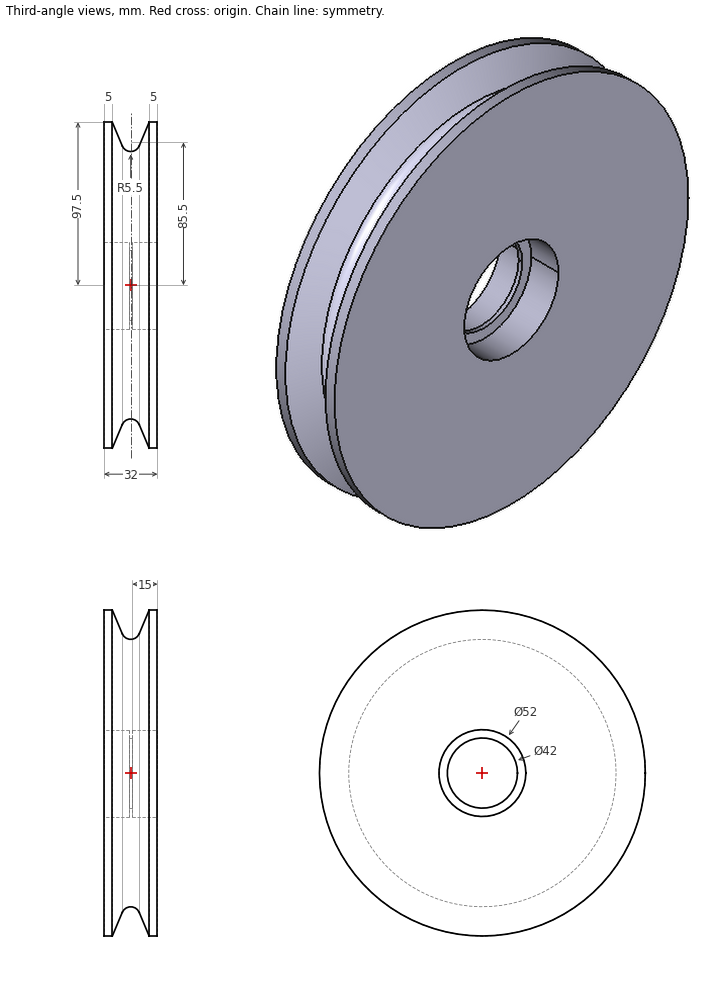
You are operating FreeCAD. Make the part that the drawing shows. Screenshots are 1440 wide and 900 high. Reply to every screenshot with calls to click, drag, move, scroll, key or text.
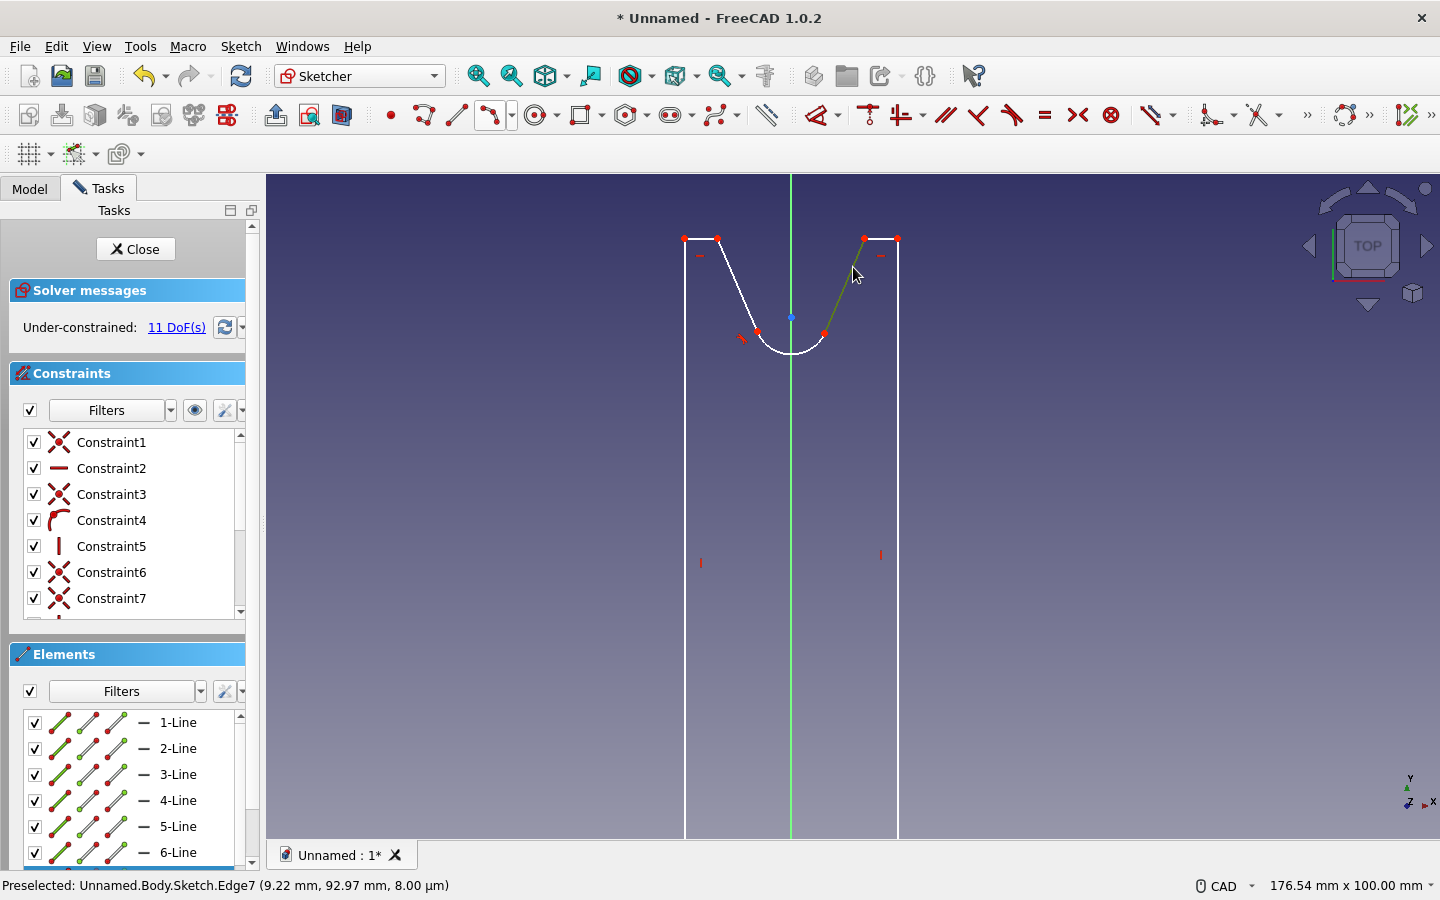
click(774, 350)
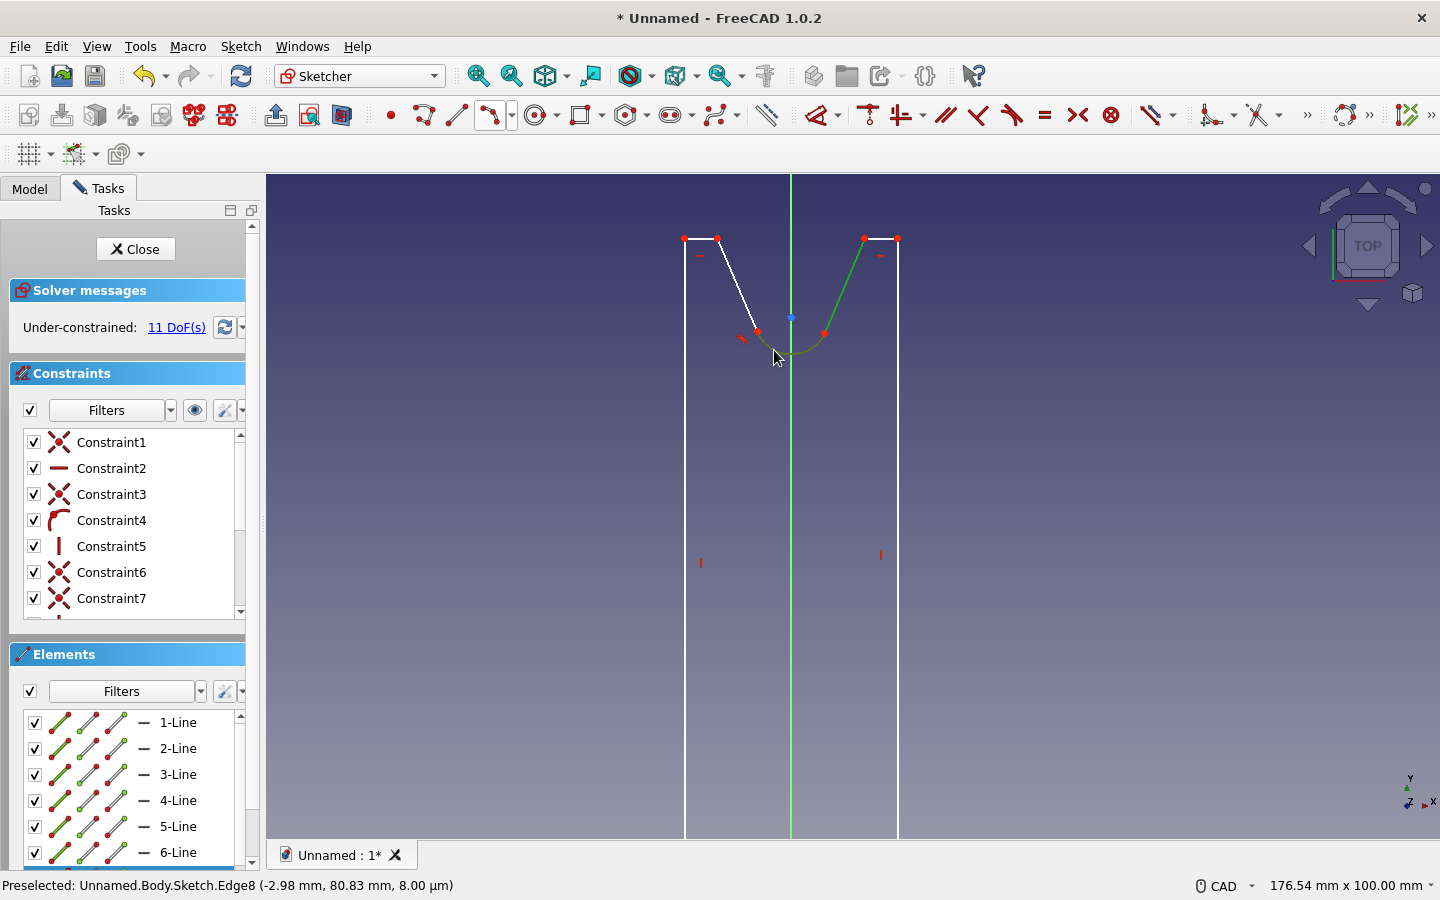
click(1012, 116)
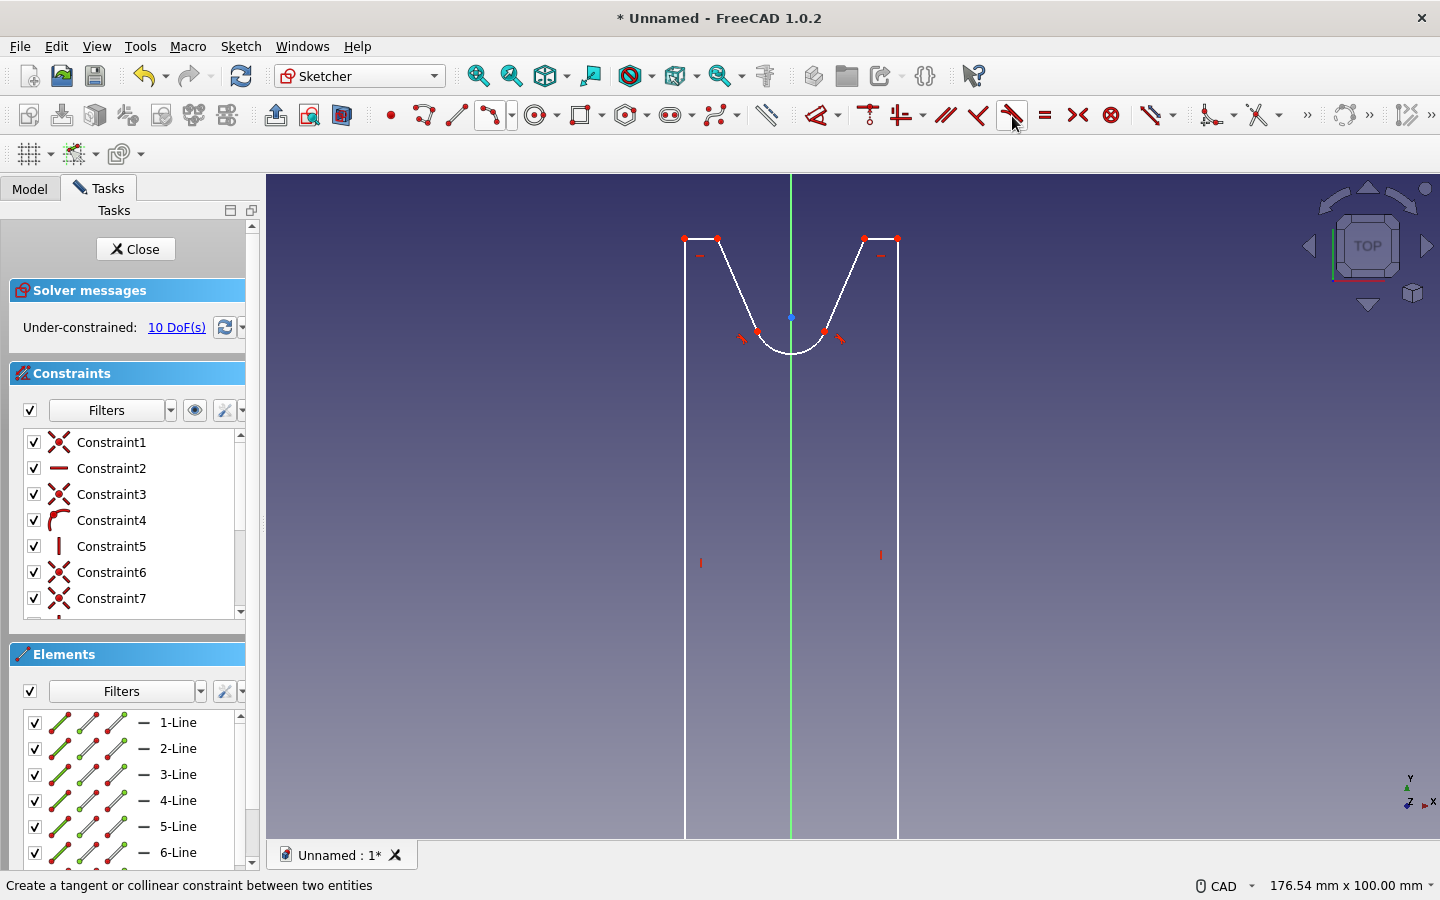
scroll(771, 394, down, 2)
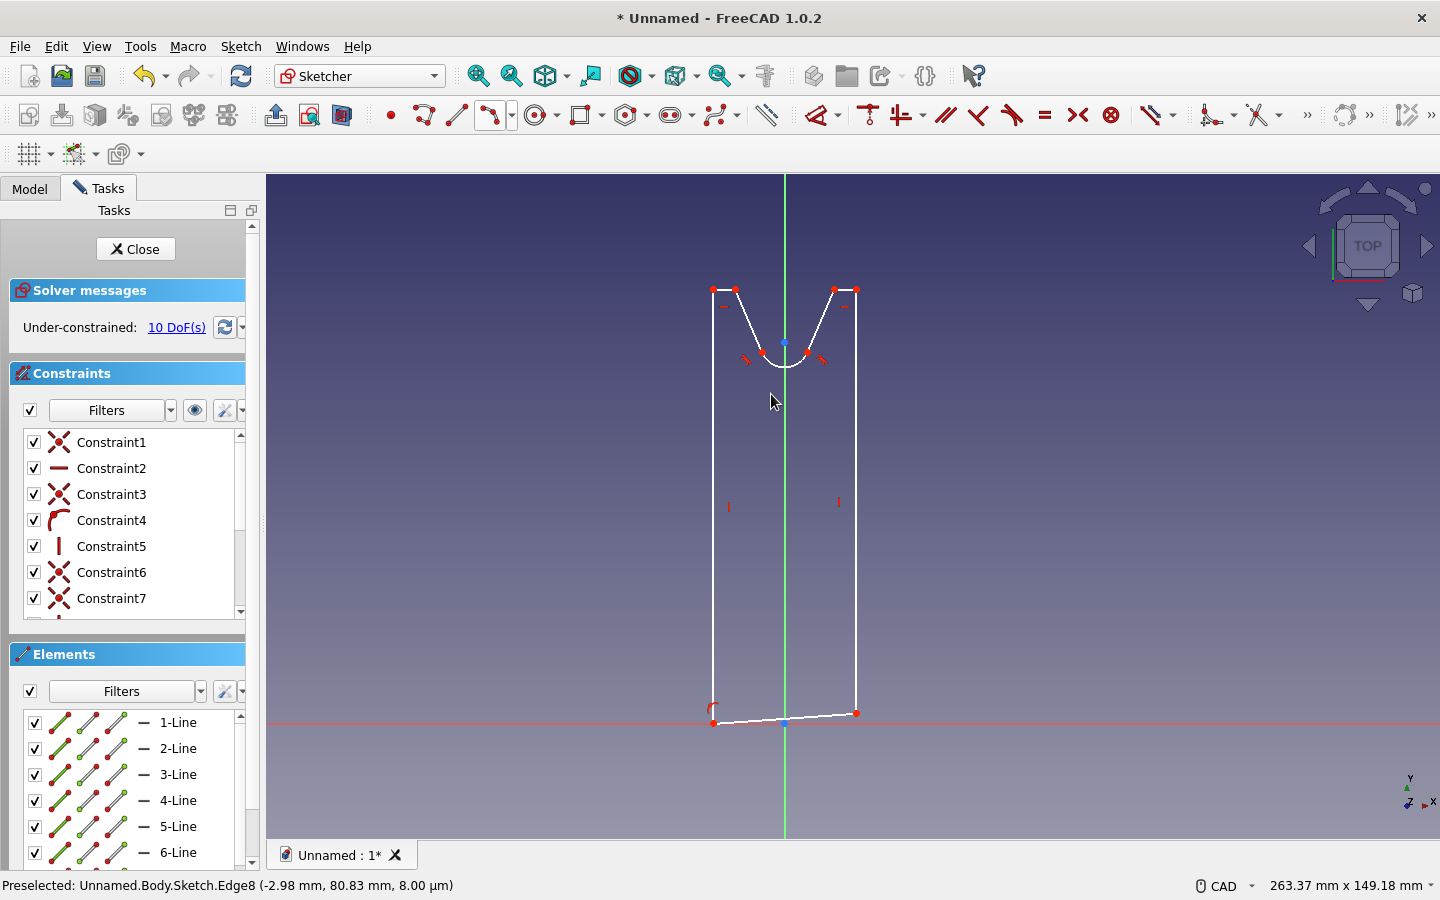
scroll(813, 717, up, 4)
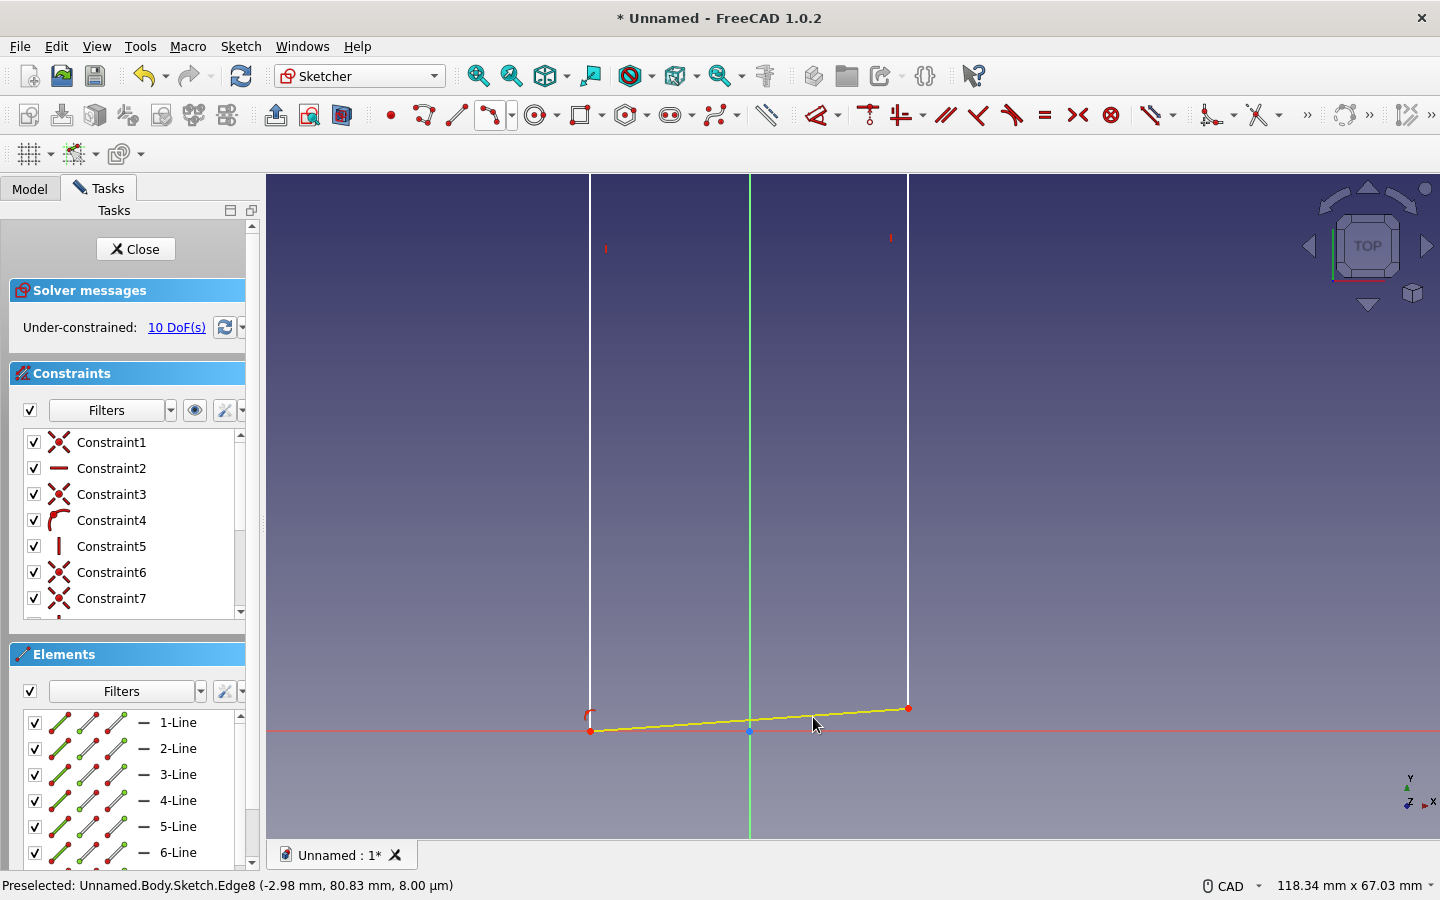
click(813, 716)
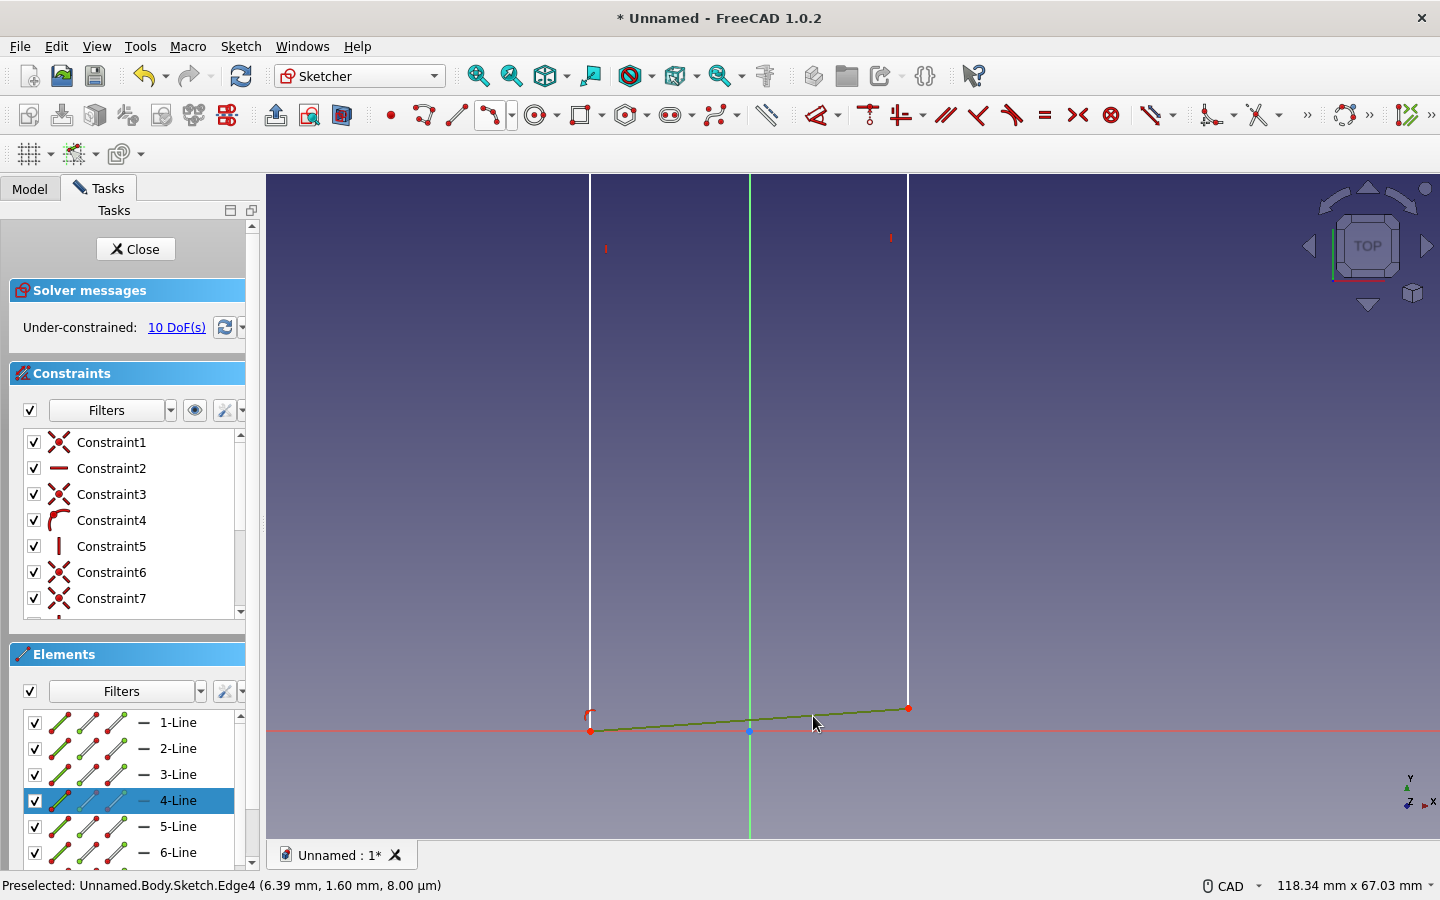
key(h)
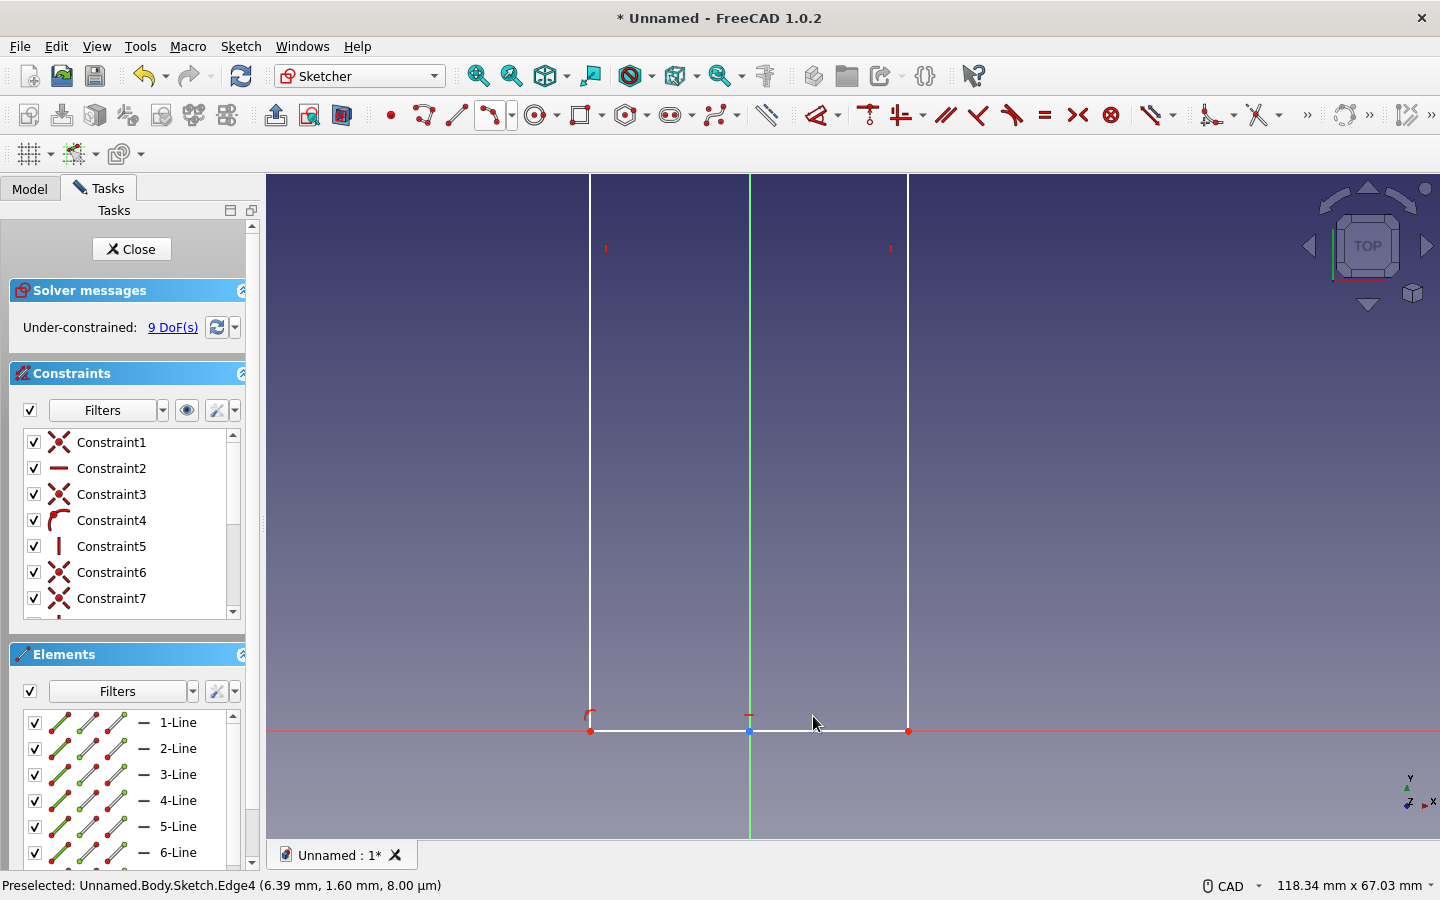
scroll(813, 718, down, 4)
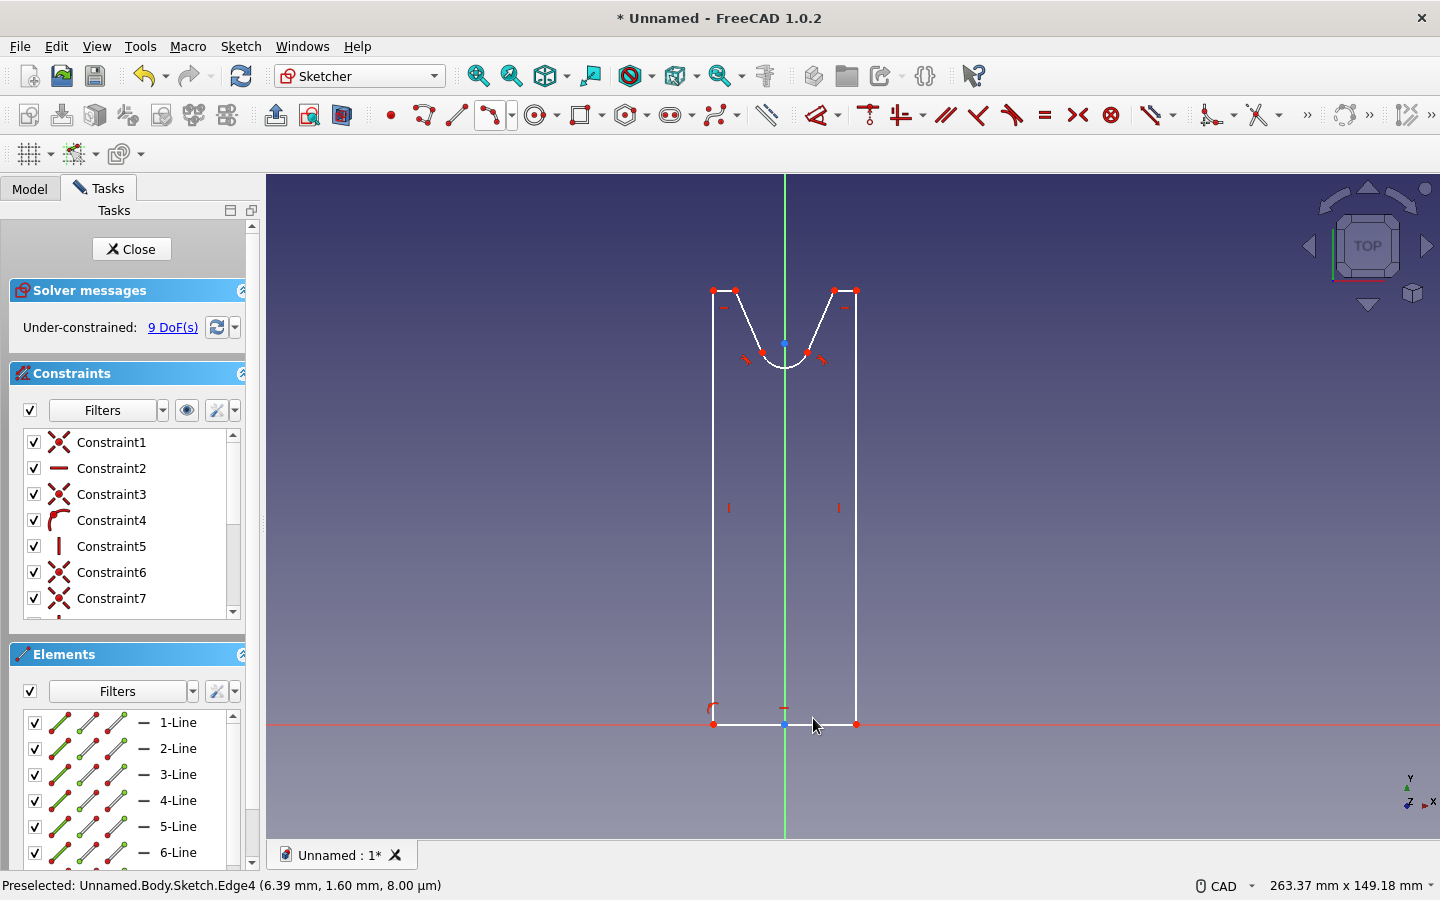
click(785, 343)